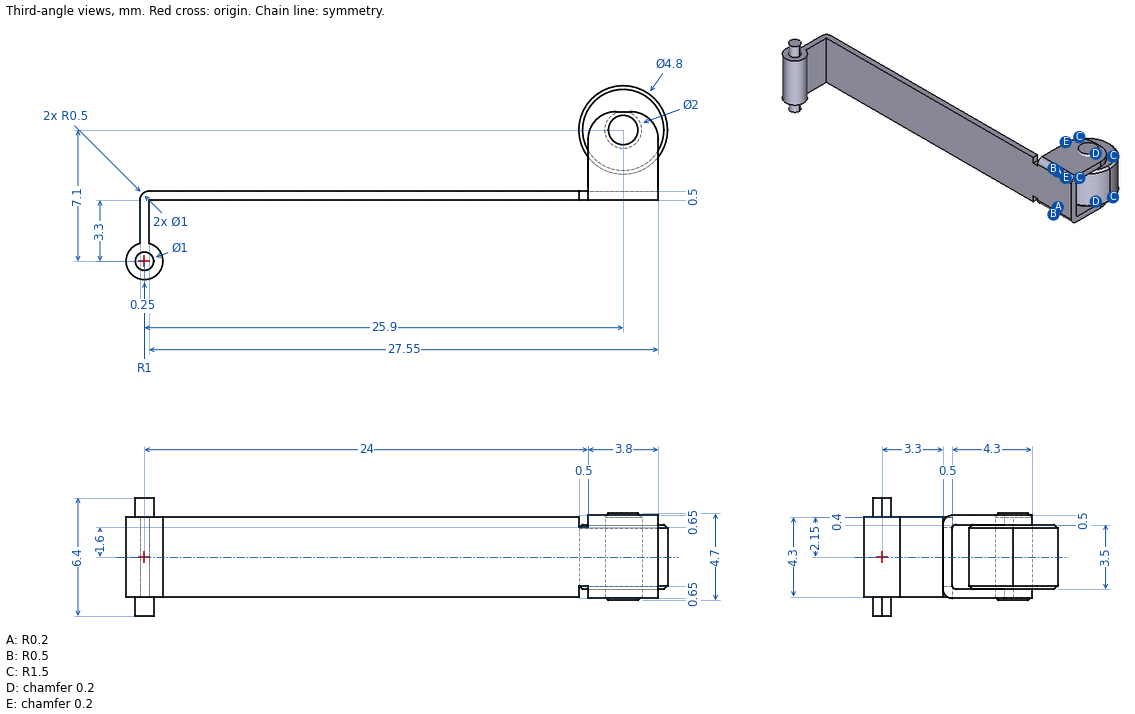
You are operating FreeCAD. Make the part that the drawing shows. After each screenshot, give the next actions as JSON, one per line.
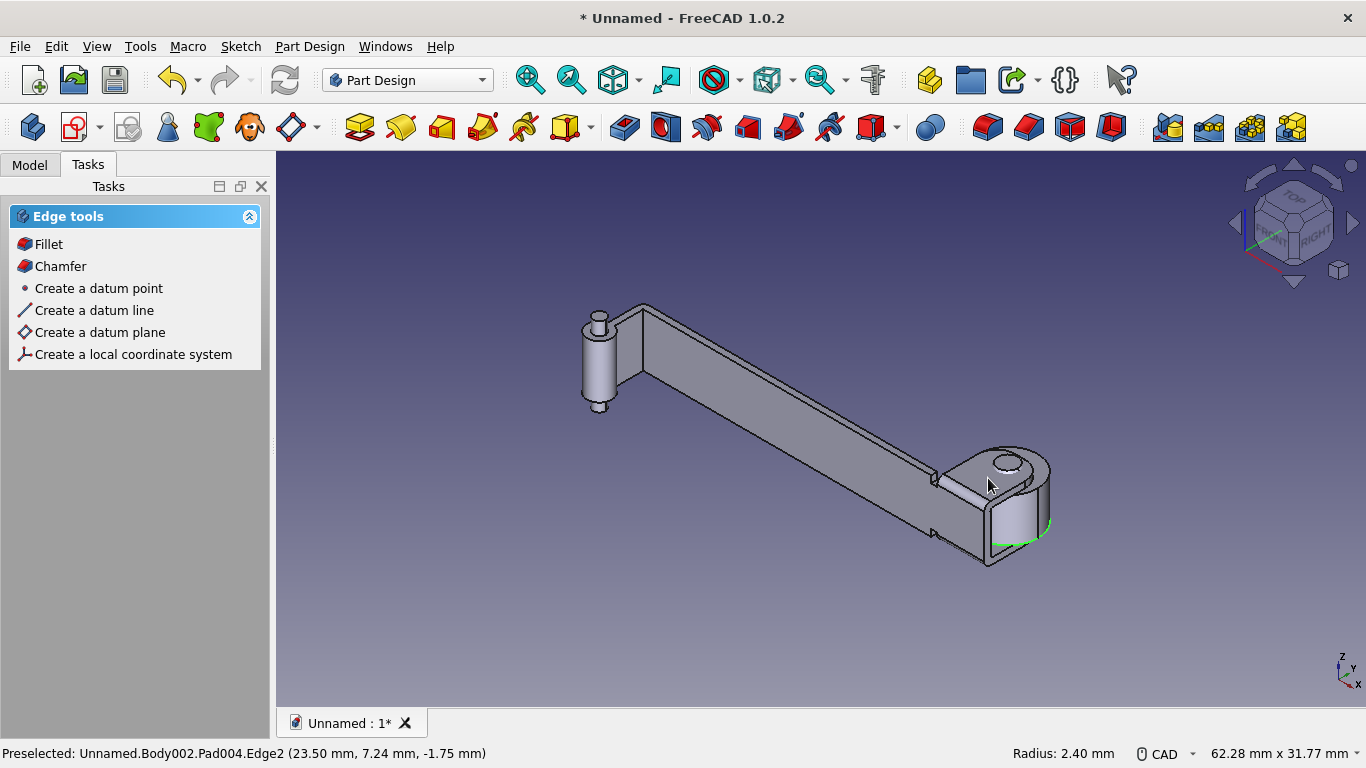
{"action": "key", "text": "v f"}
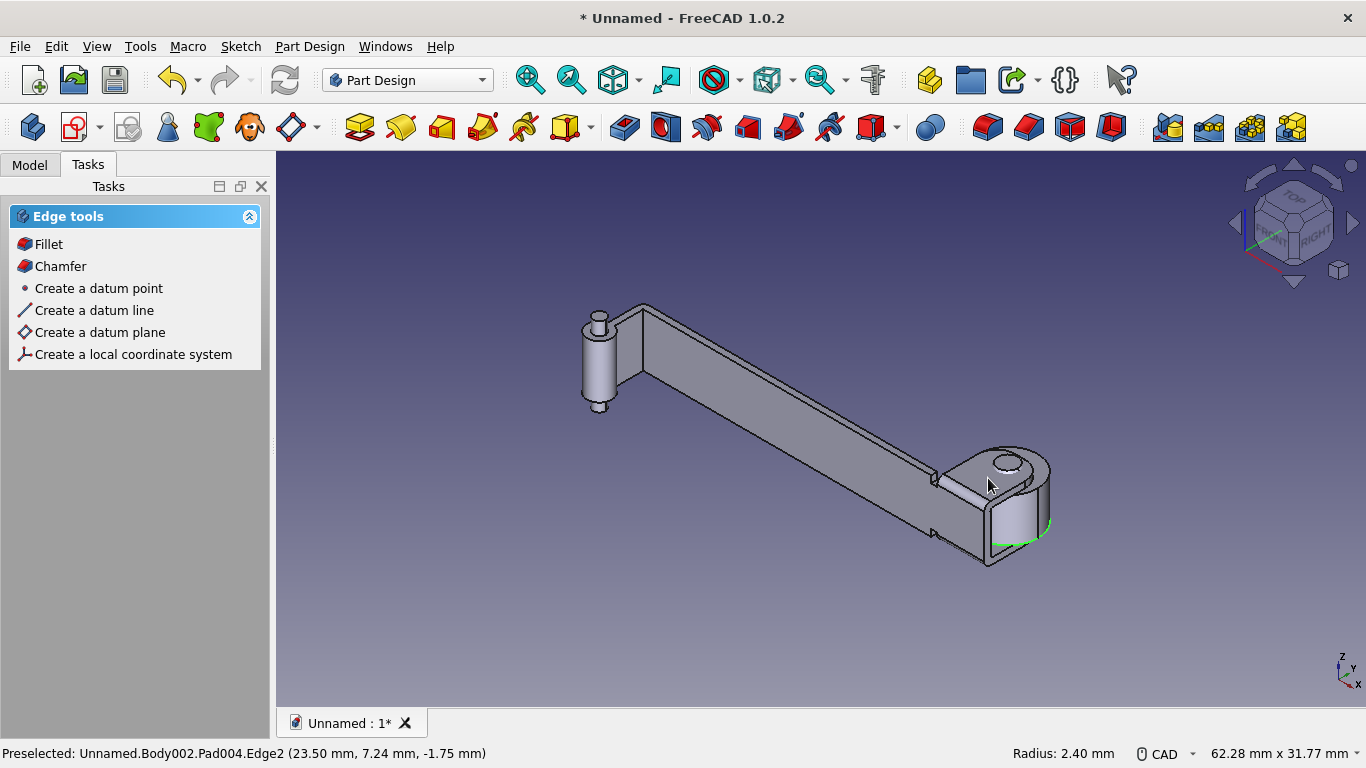
{"action": "left_click", "coordinate": [1045, 459], "text": "ctrl"}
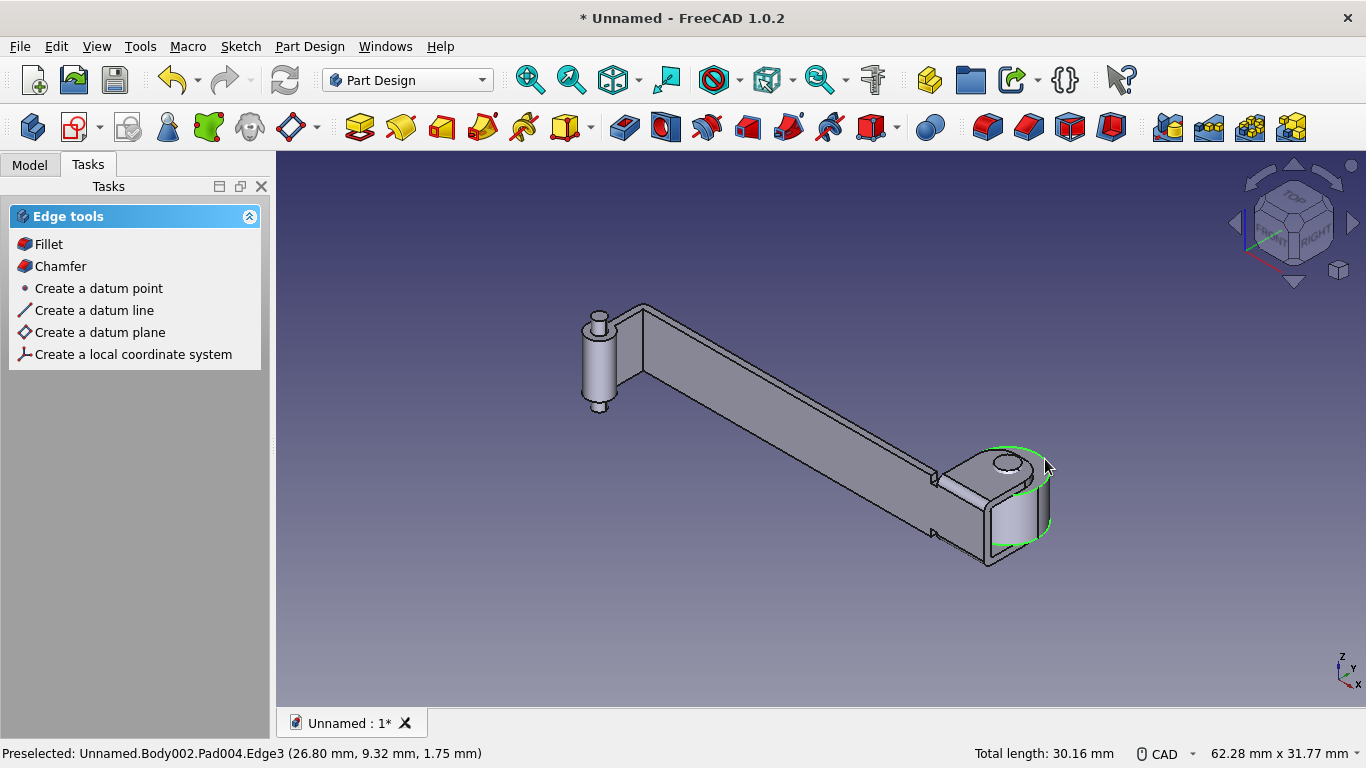
{"action": "left_click", "coordinate": [1029, 128]}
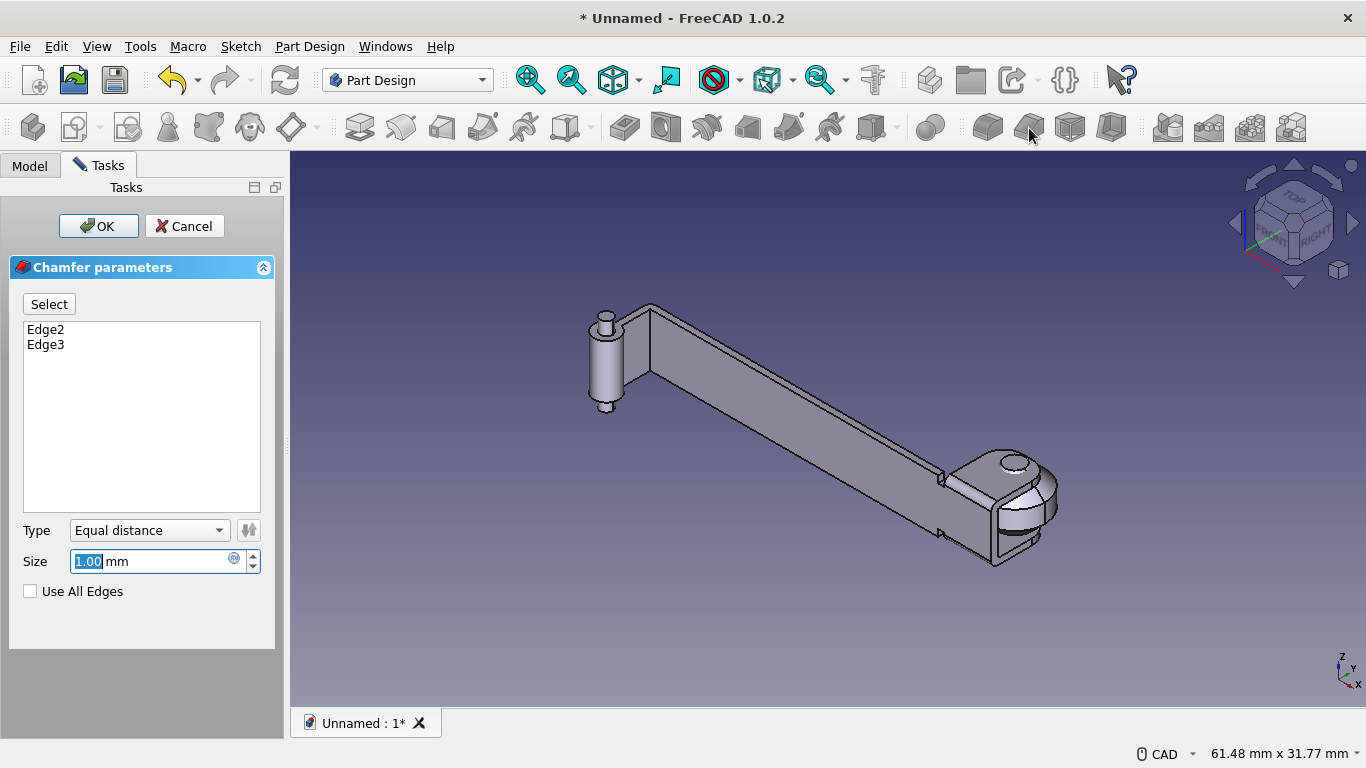
{"action": "type", "text": "0.2"}
{"action": "key", "text": "Tab"}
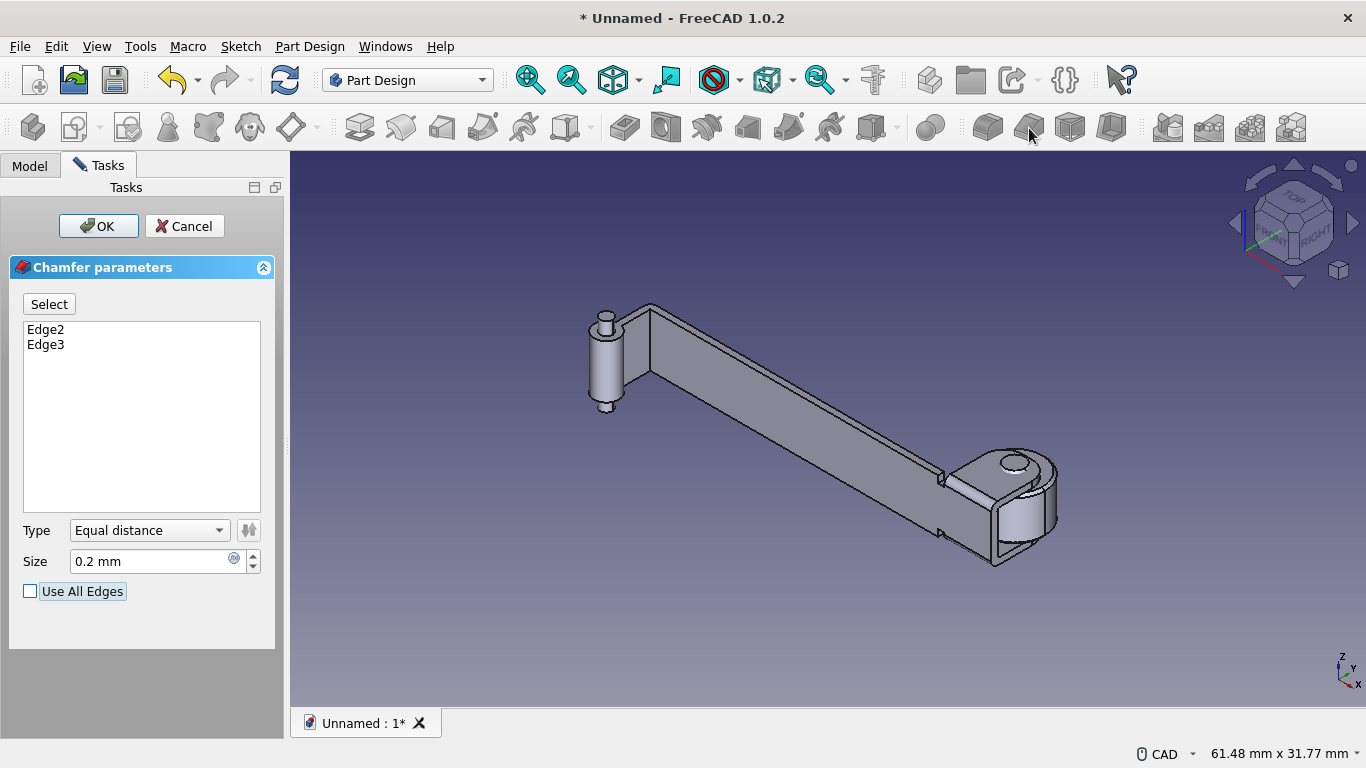
{"action": "left_click", "coordinate": [99, 226]}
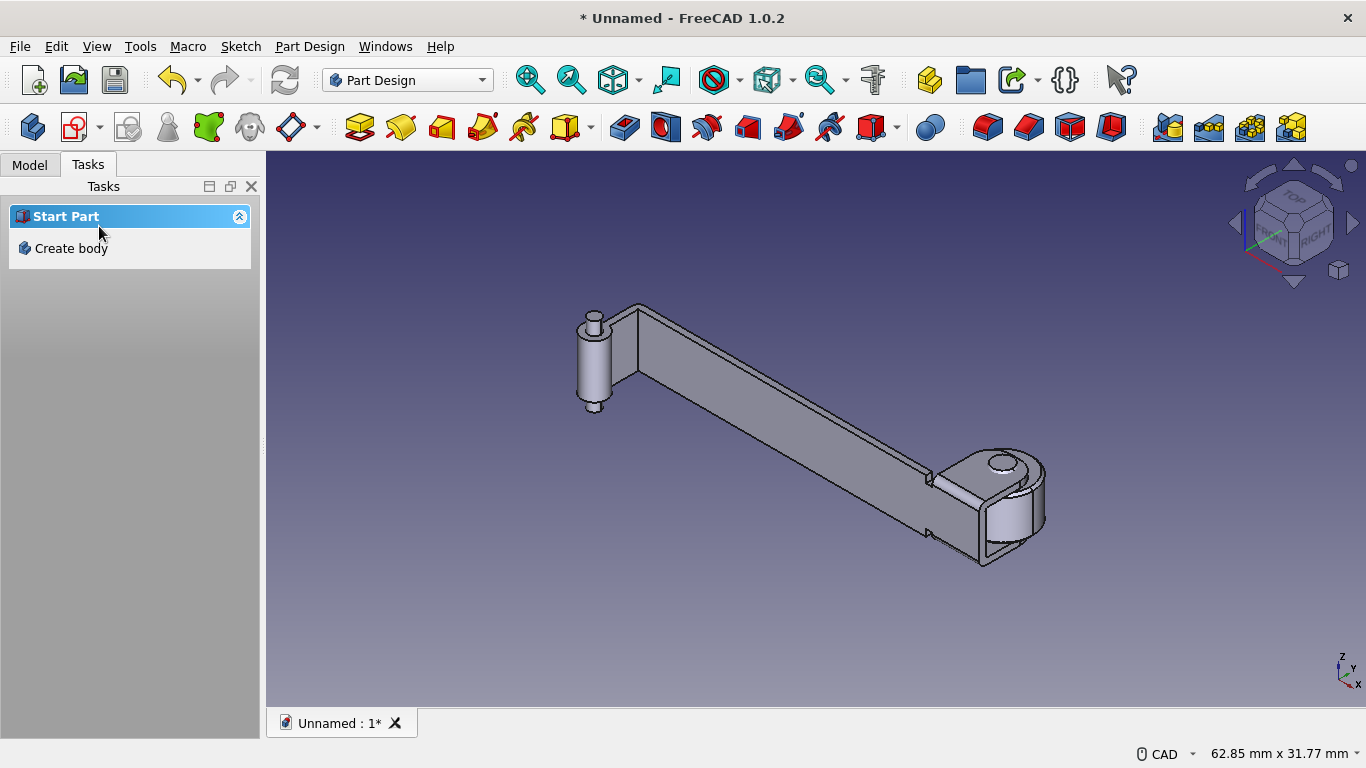
{"action": "left_click", "coordinate": [531, 80]}